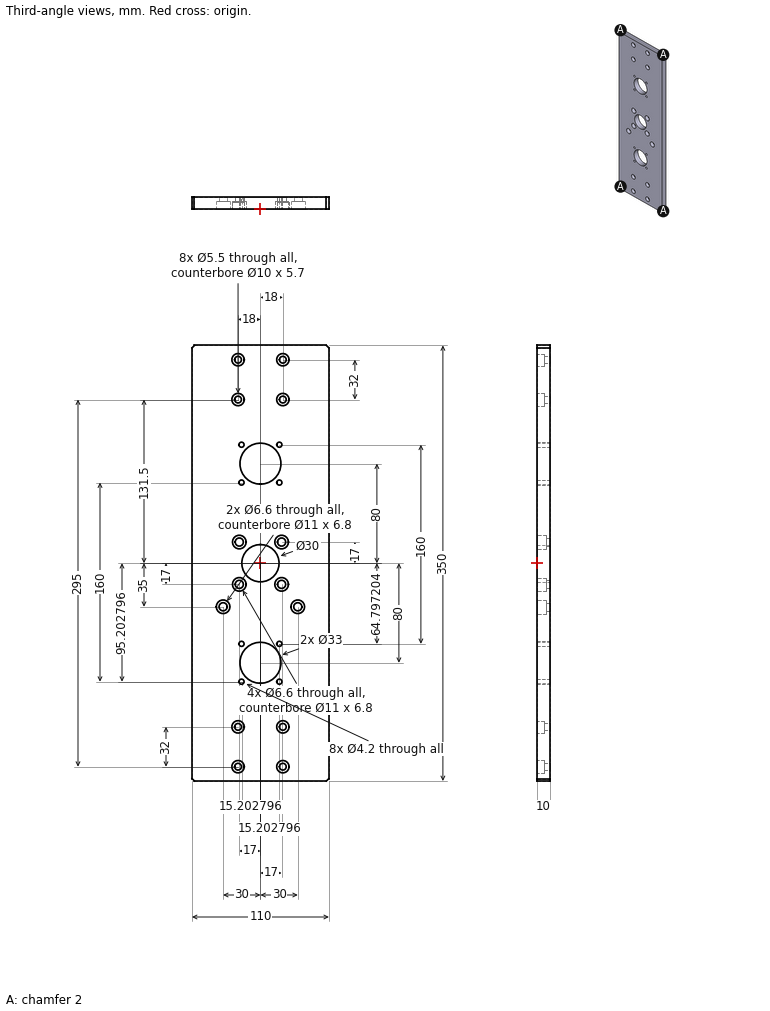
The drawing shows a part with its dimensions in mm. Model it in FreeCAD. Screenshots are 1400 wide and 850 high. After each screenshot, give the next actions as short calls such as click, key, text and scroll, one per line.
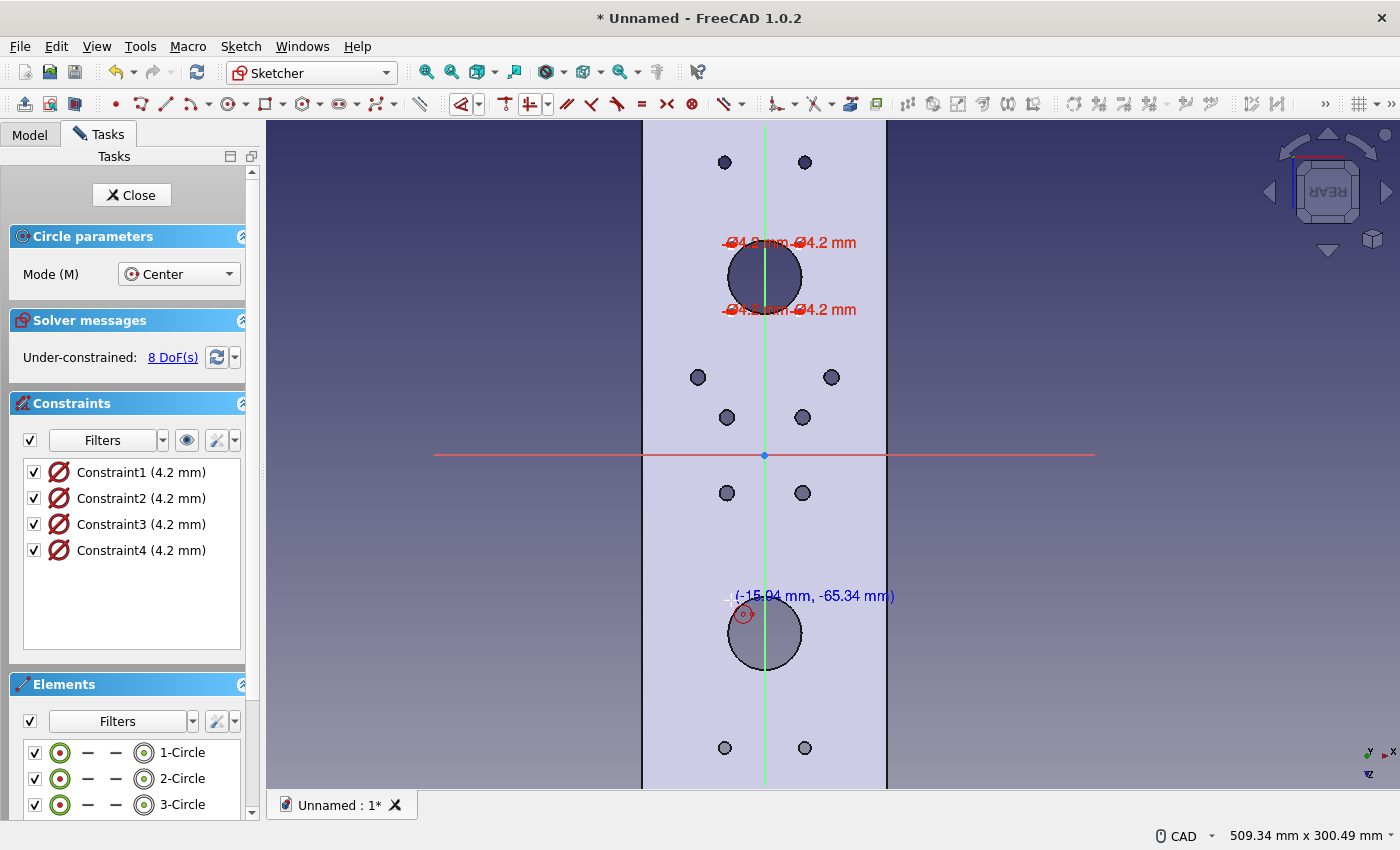
click(731, 600)
move(734, 596)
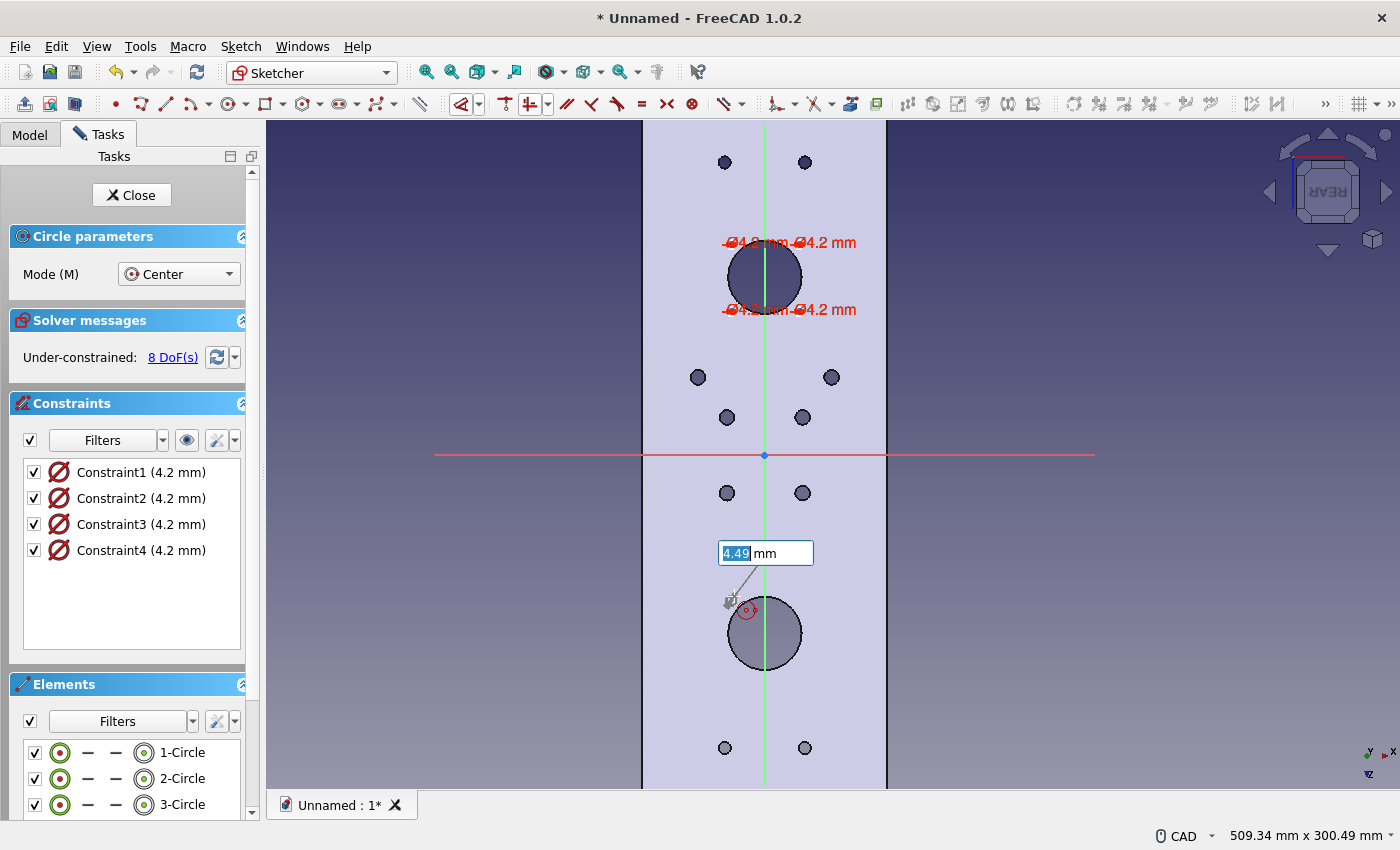
text(4.2)
key(Return)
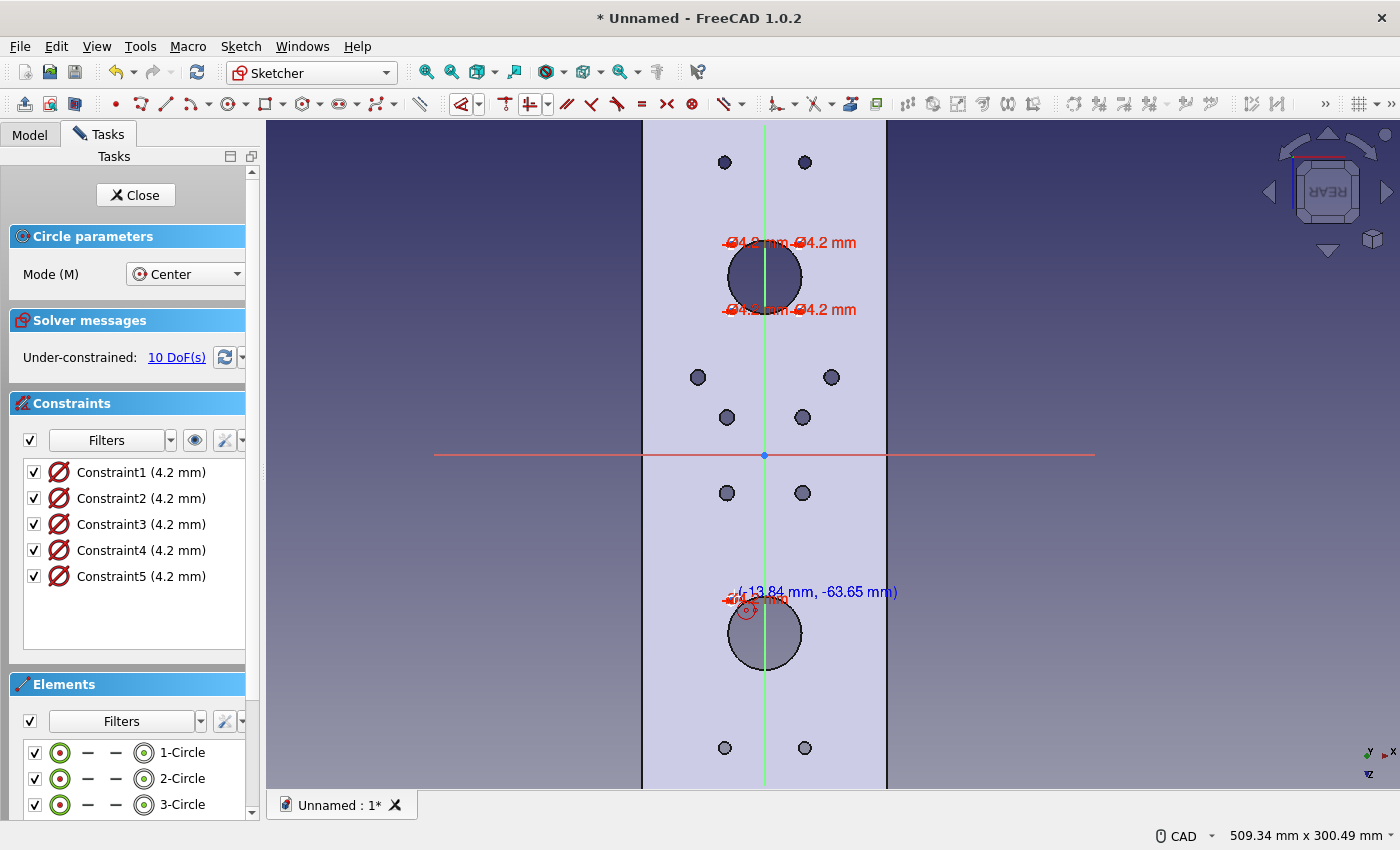
scroll(799, 667, up, 8)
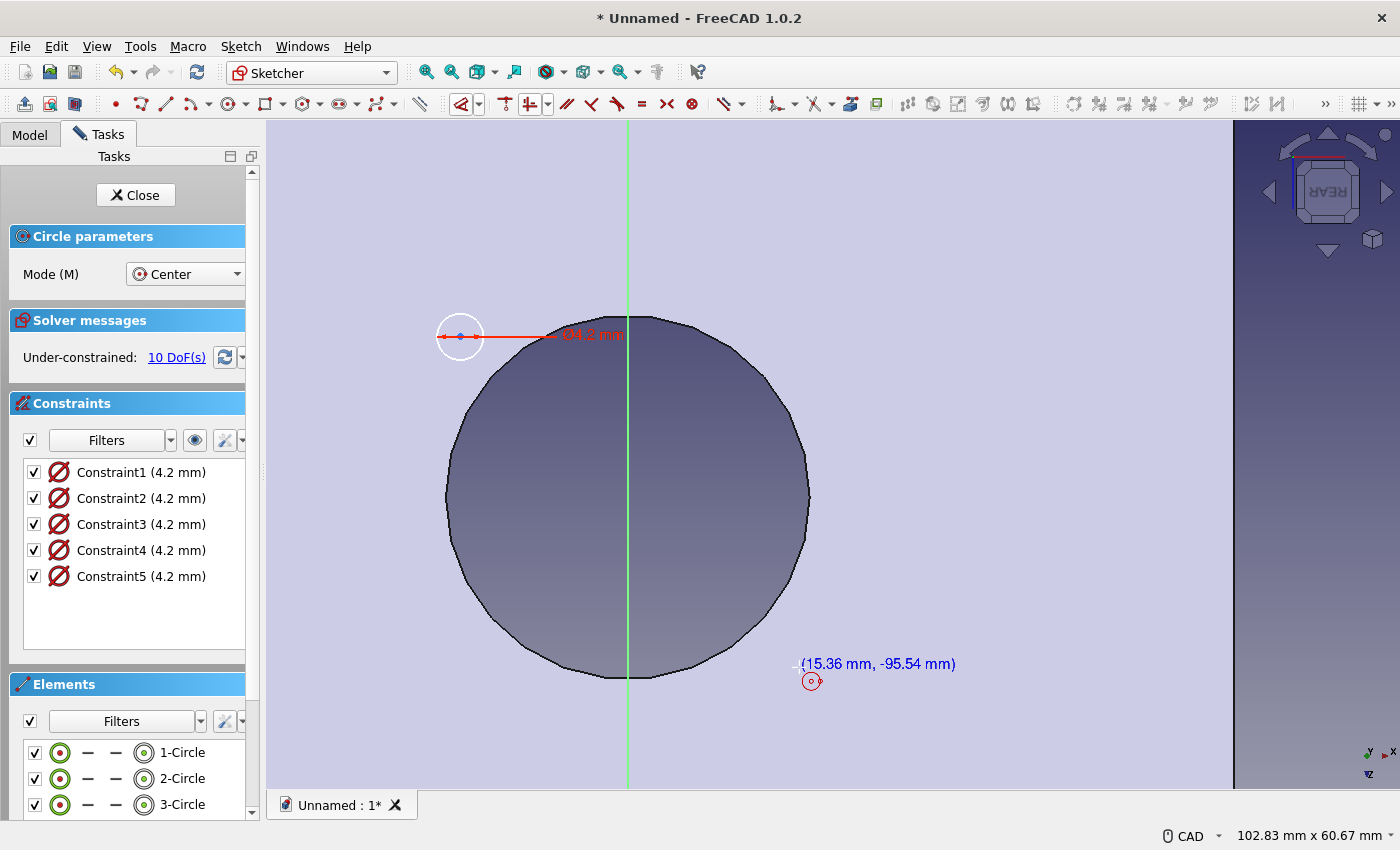
scroll(799, 667, down, 8)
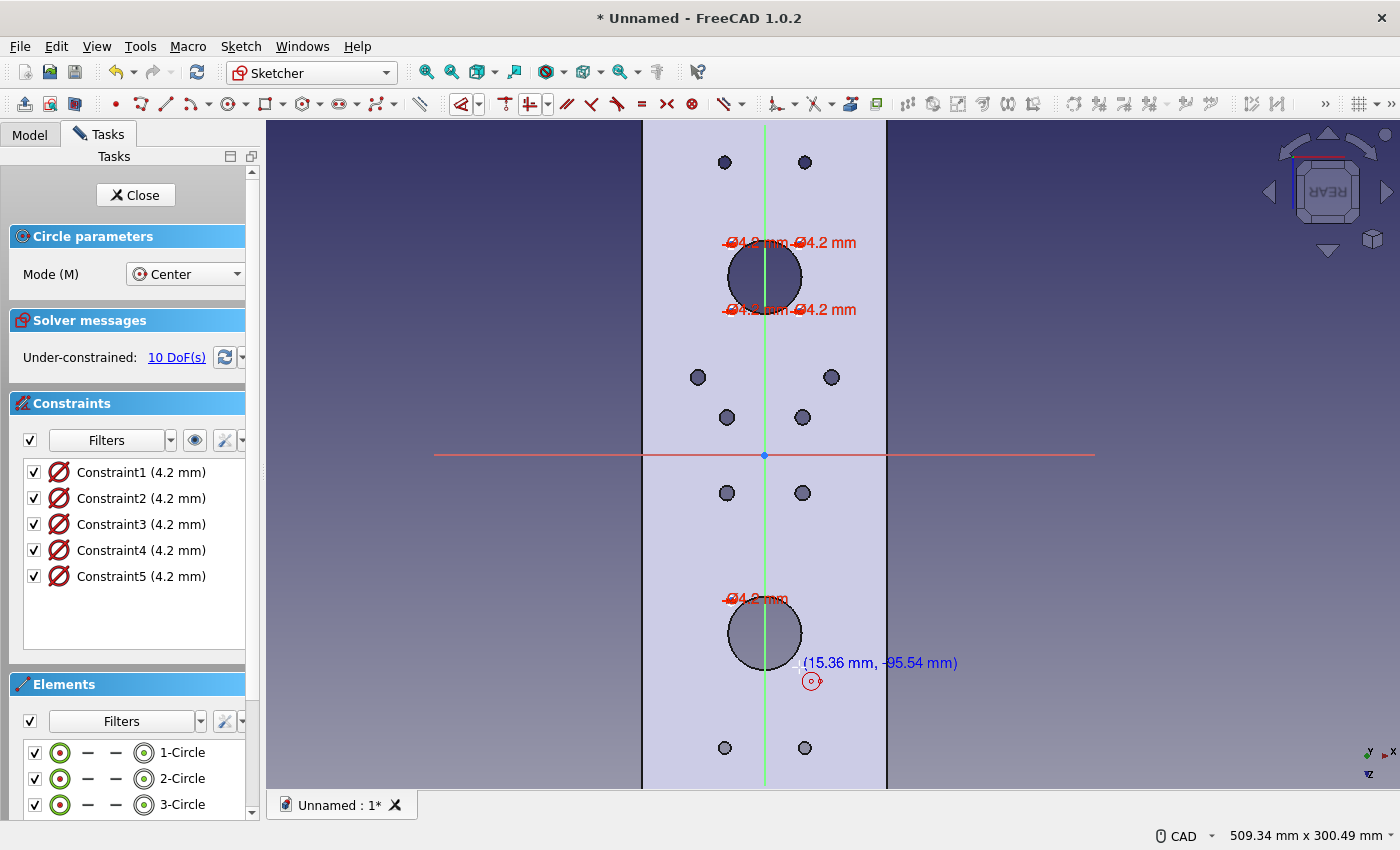
click(799, 667)
move(802, 664)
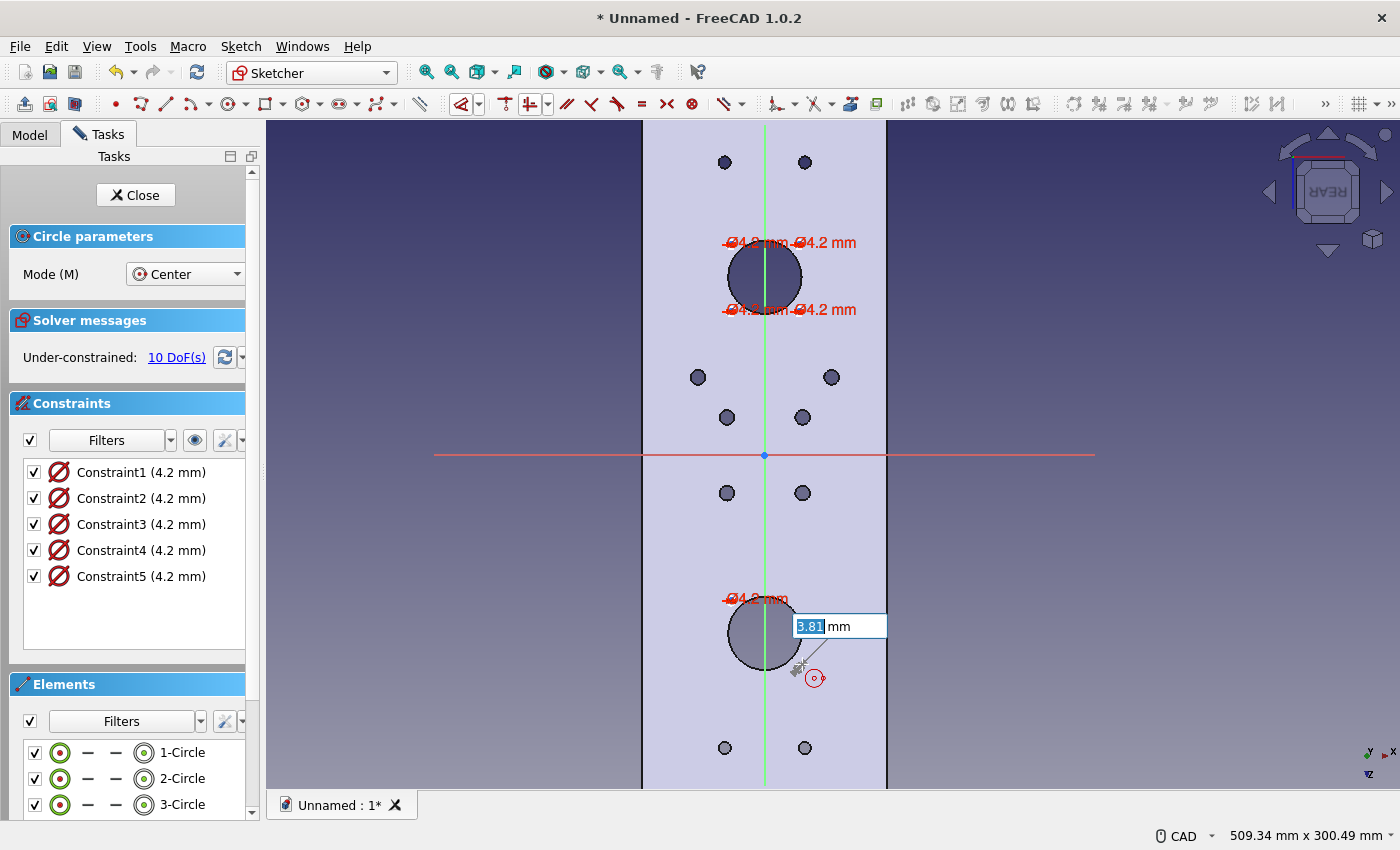
text(4.2)
key(Return)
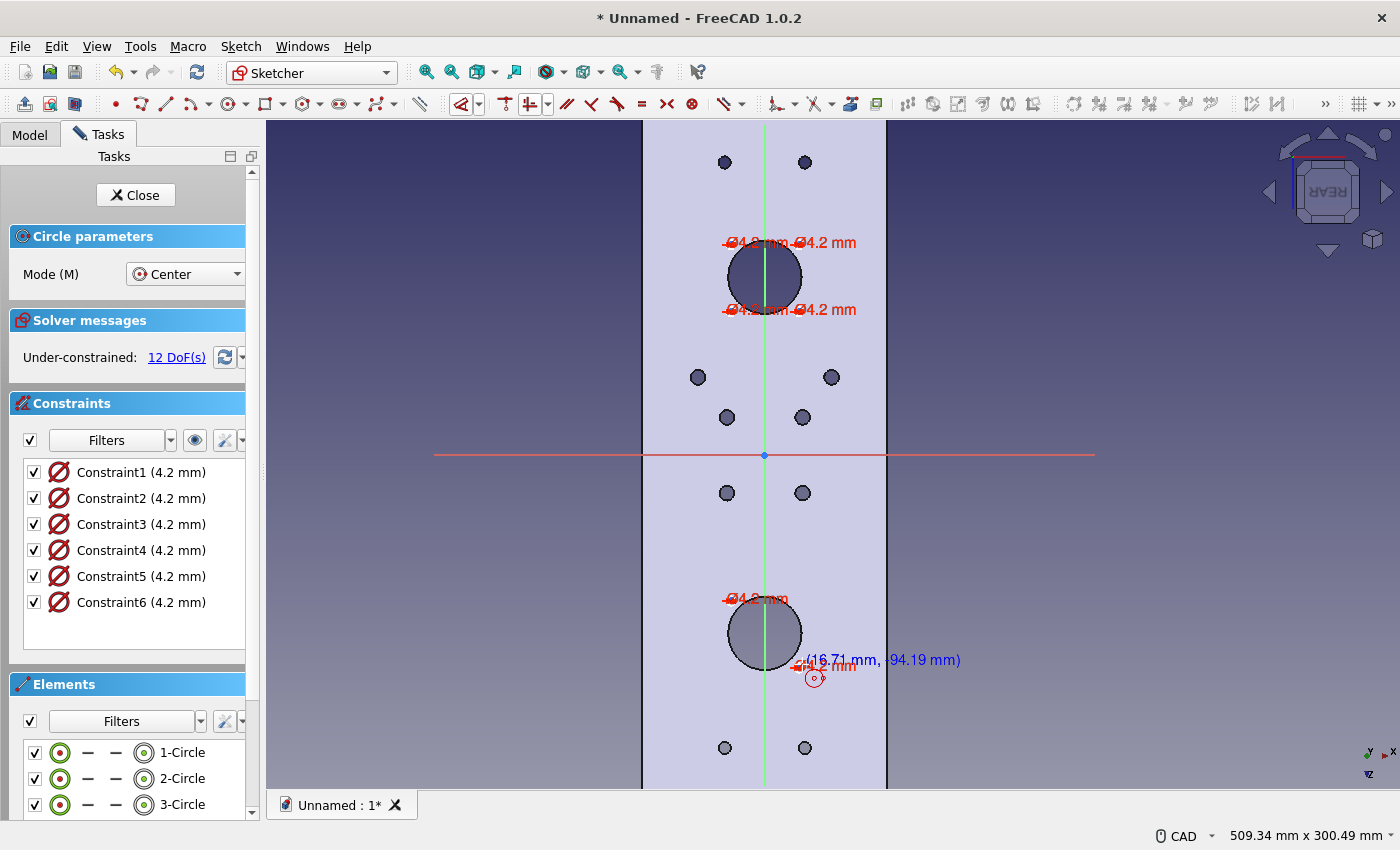
scroll(799, 600, up, 8)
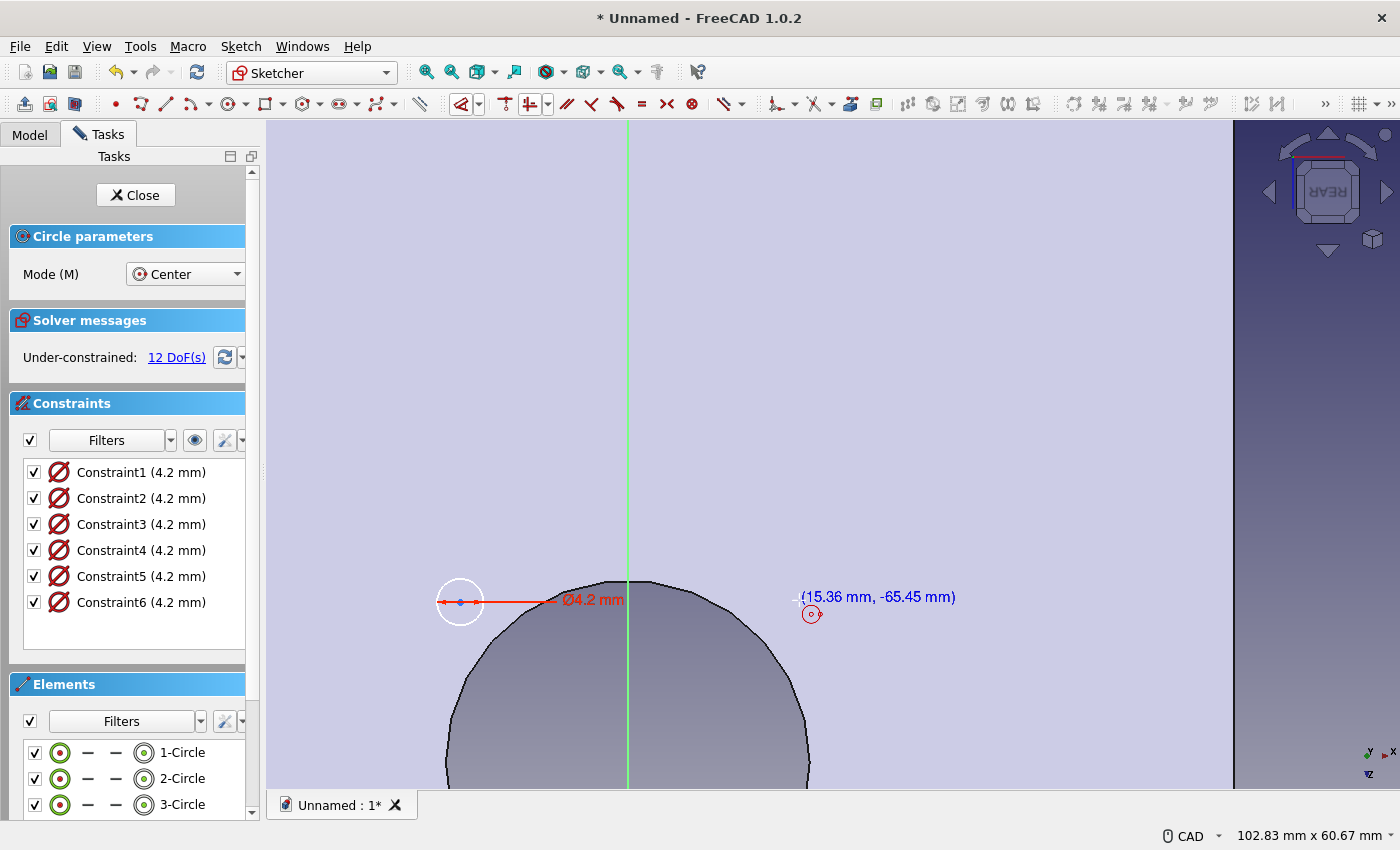
scroll(799, 600, down, 8)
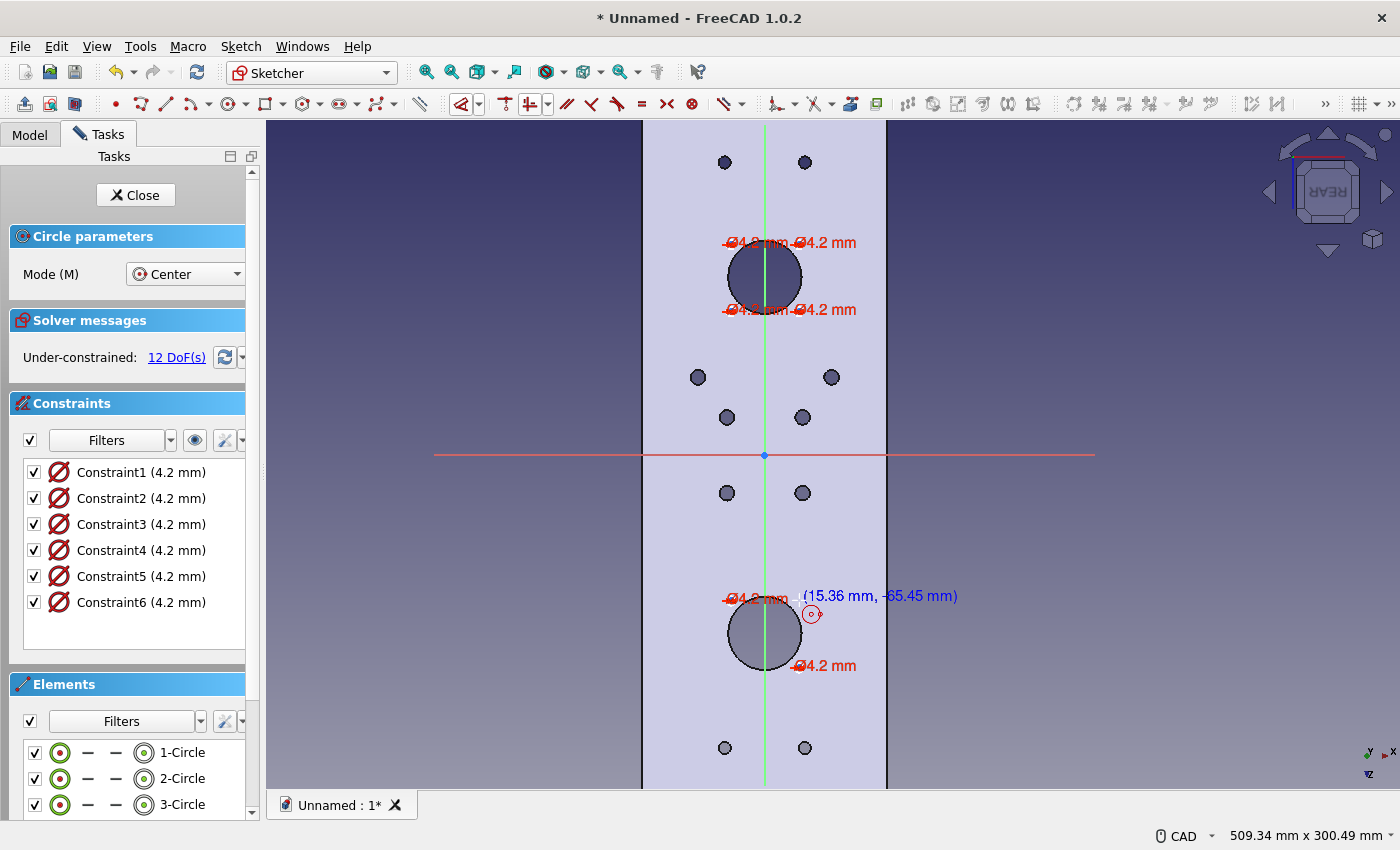
click(799, 600)
move(802, 596)